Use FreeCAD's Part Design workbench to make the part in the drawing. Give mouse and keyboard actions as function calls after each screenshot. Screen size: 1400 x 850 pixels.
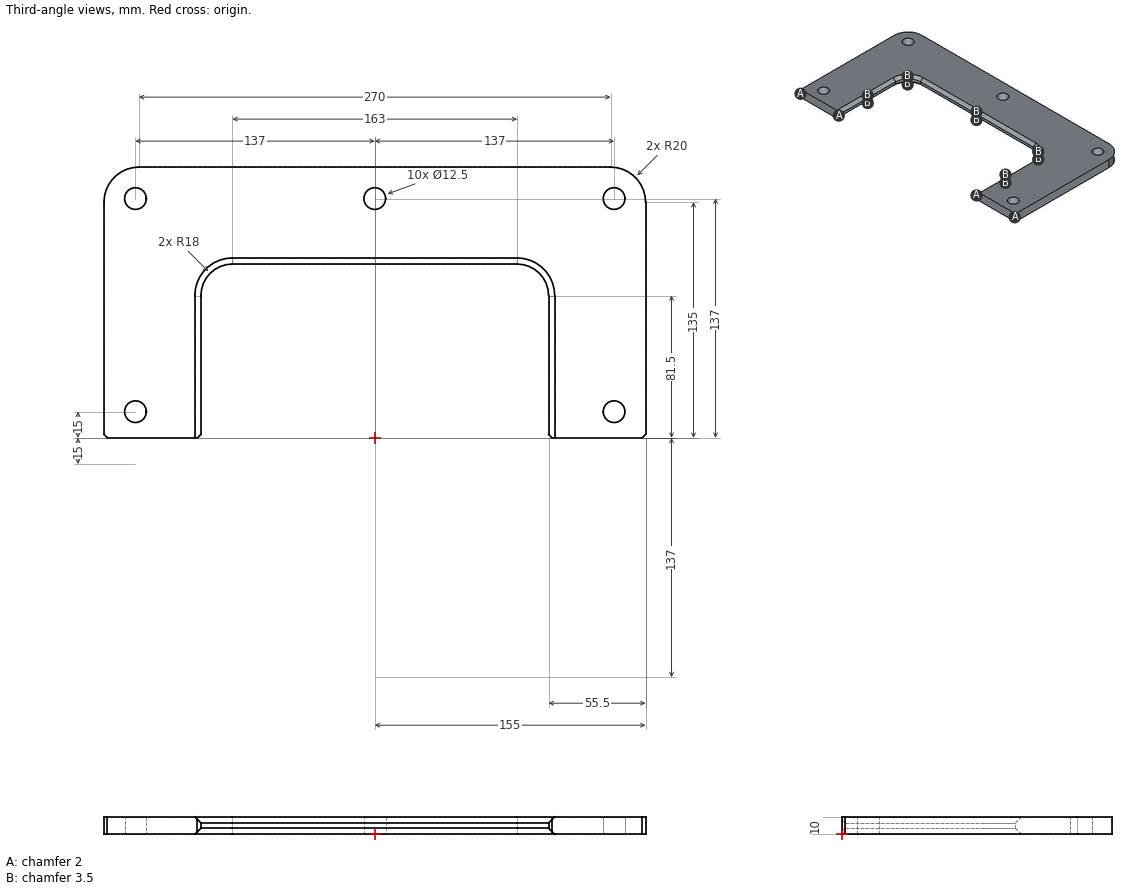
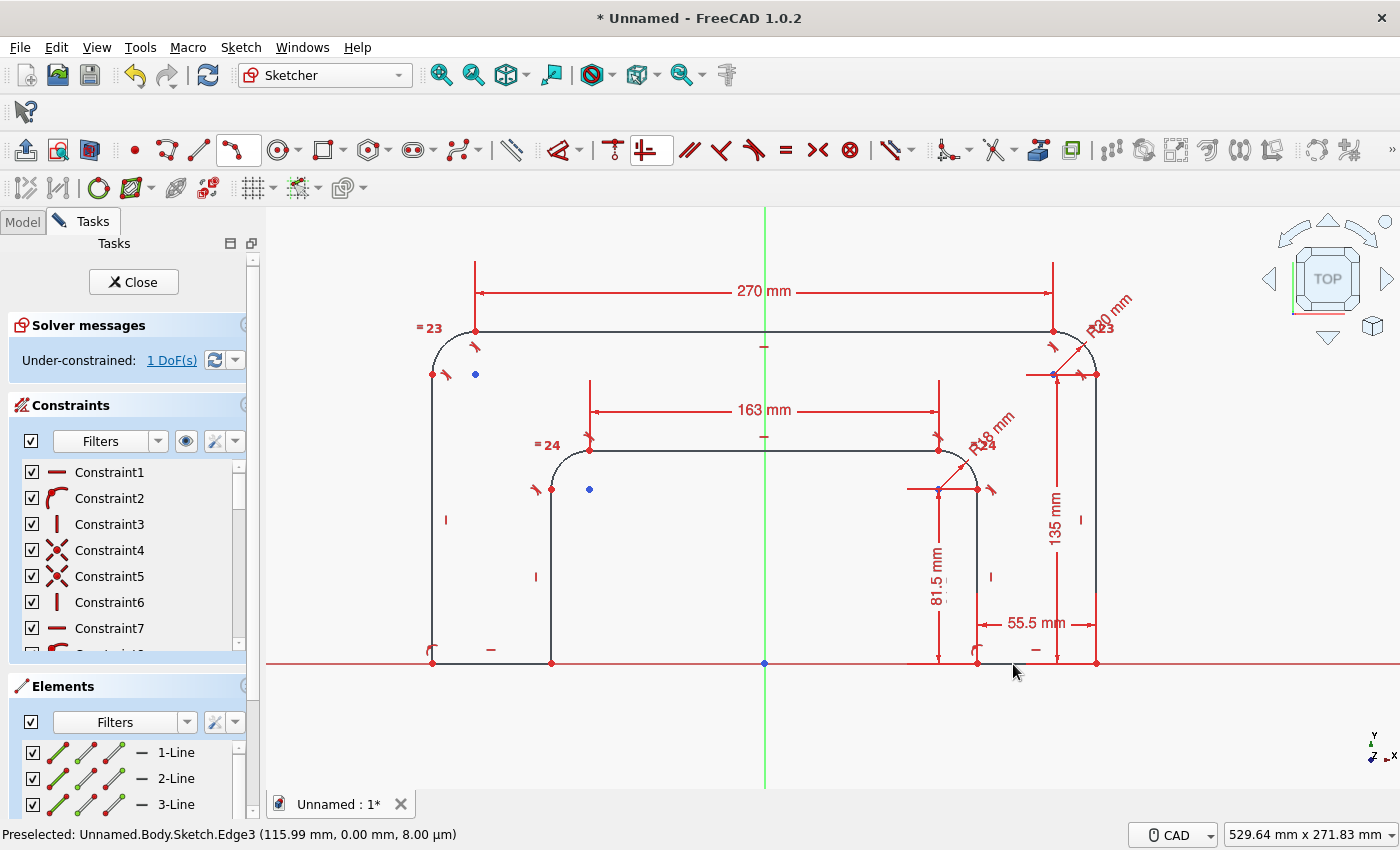
click(1096, 664)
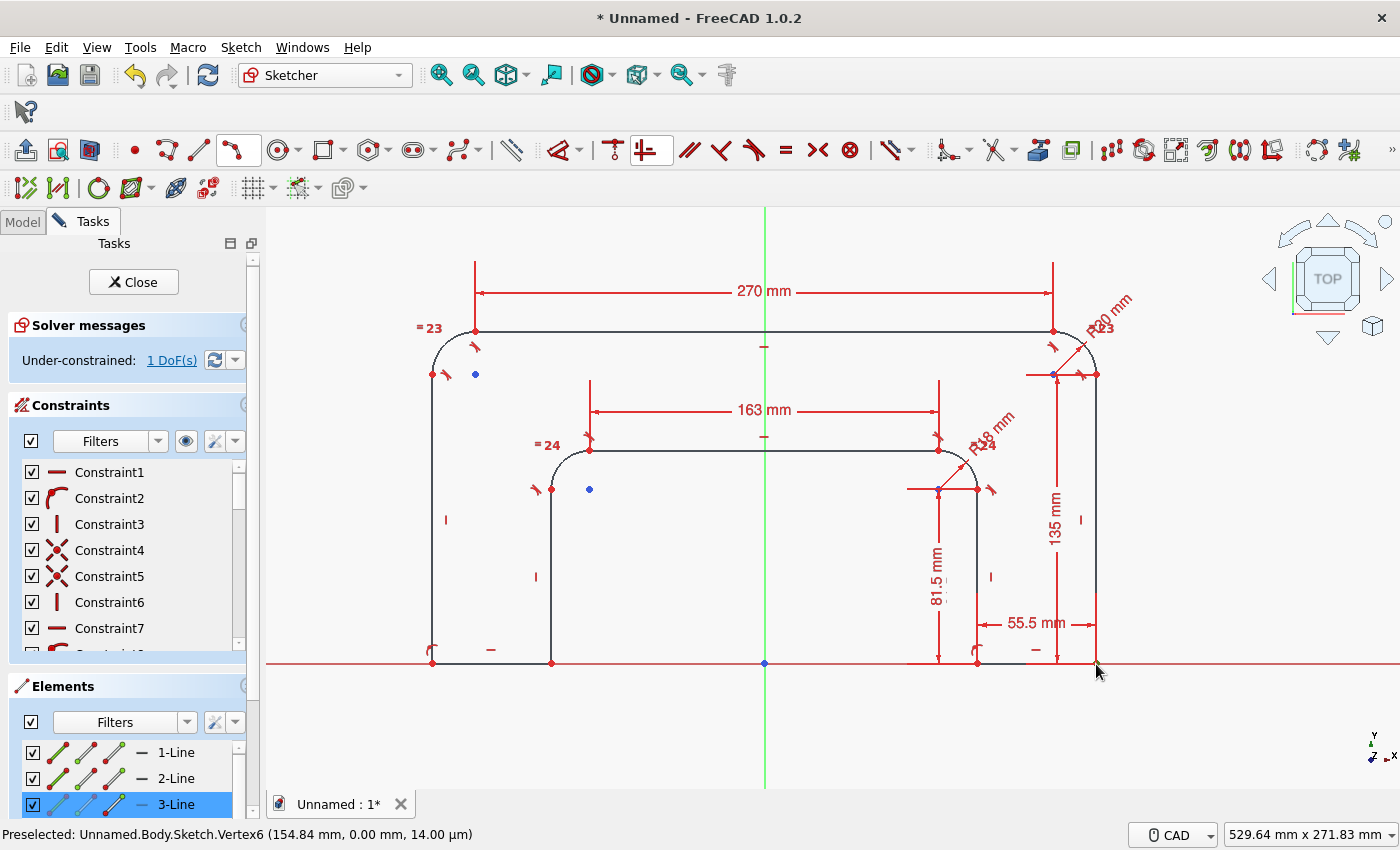
key(l)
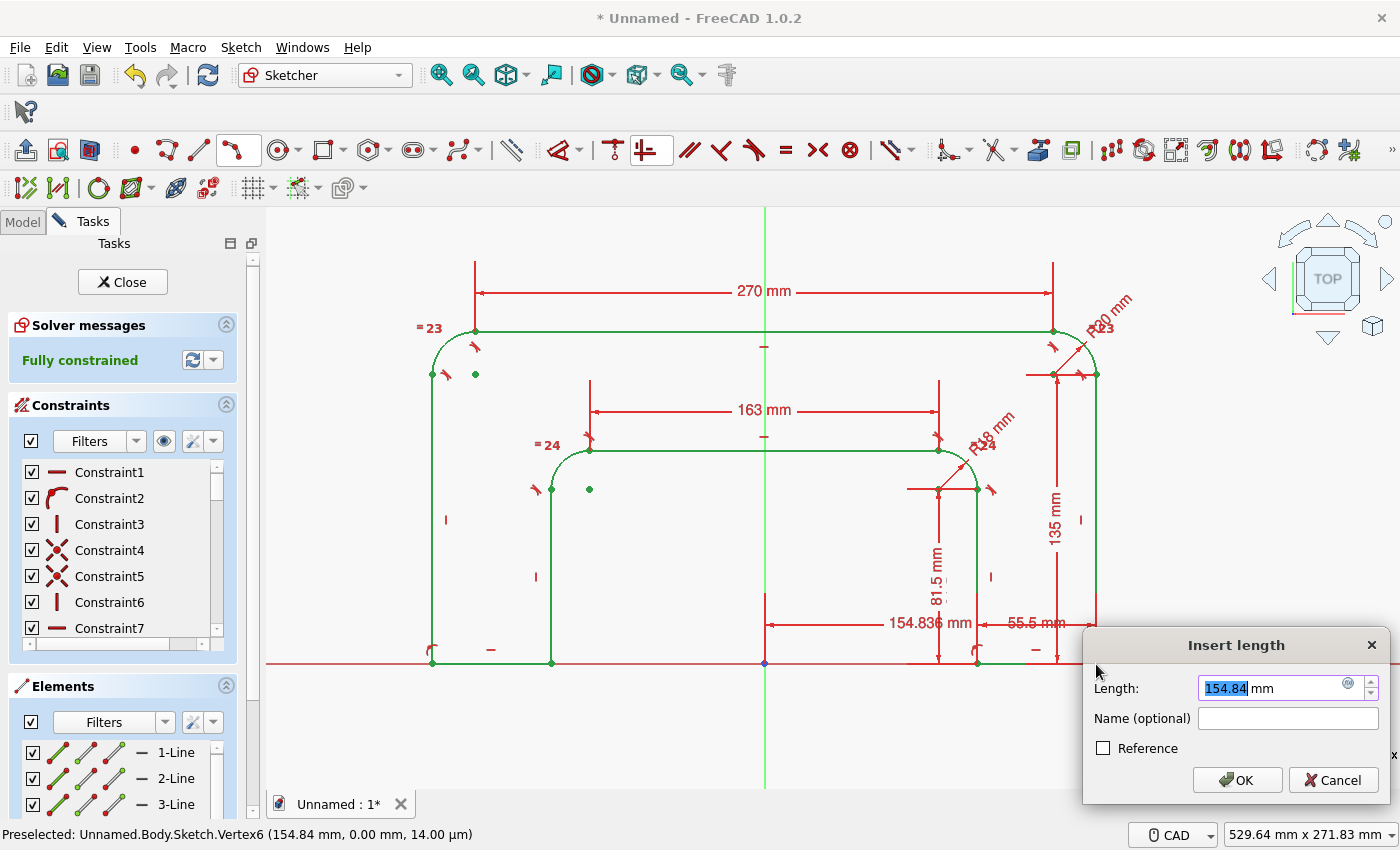
text(155)
key(Return)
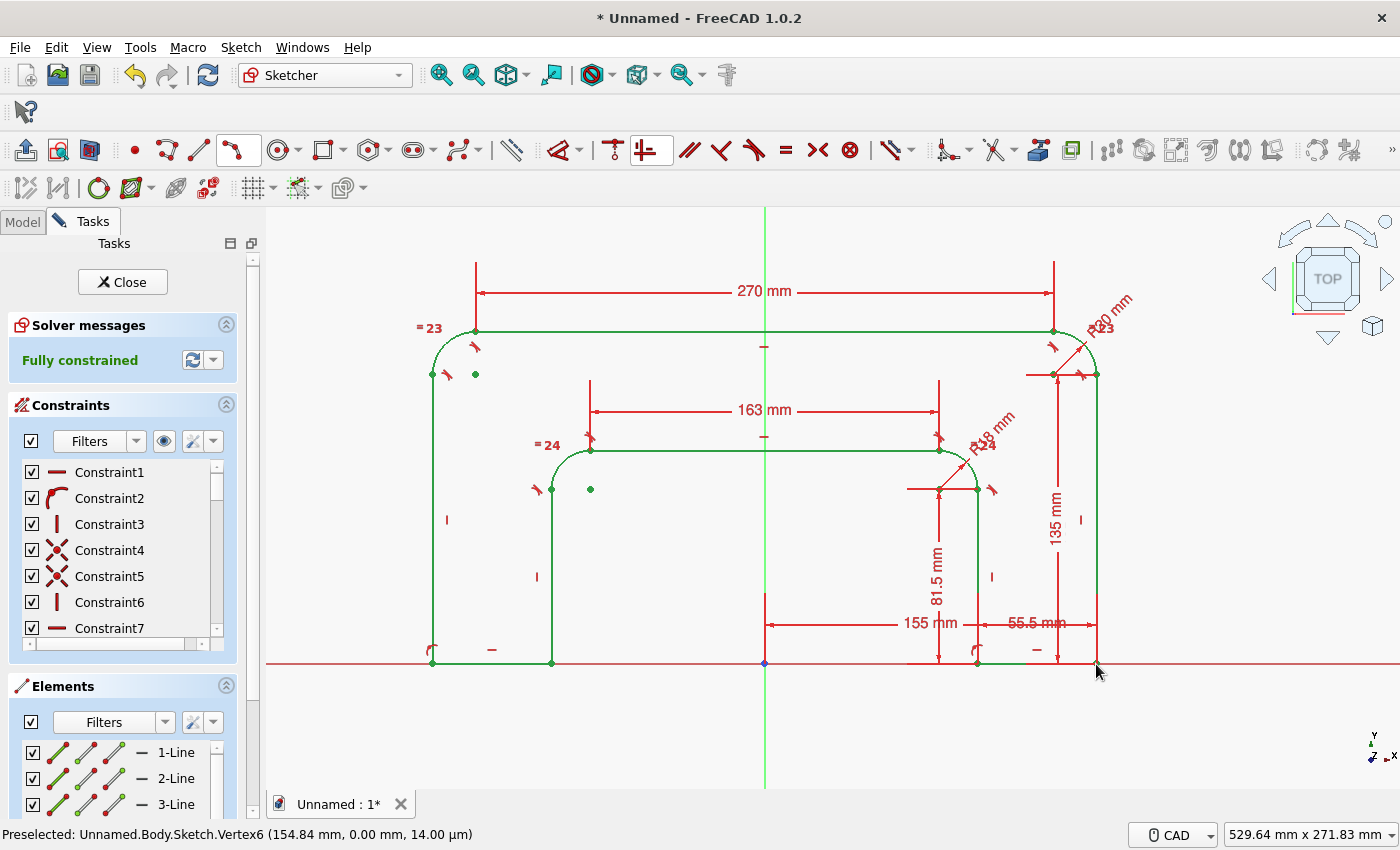
click(123, 282)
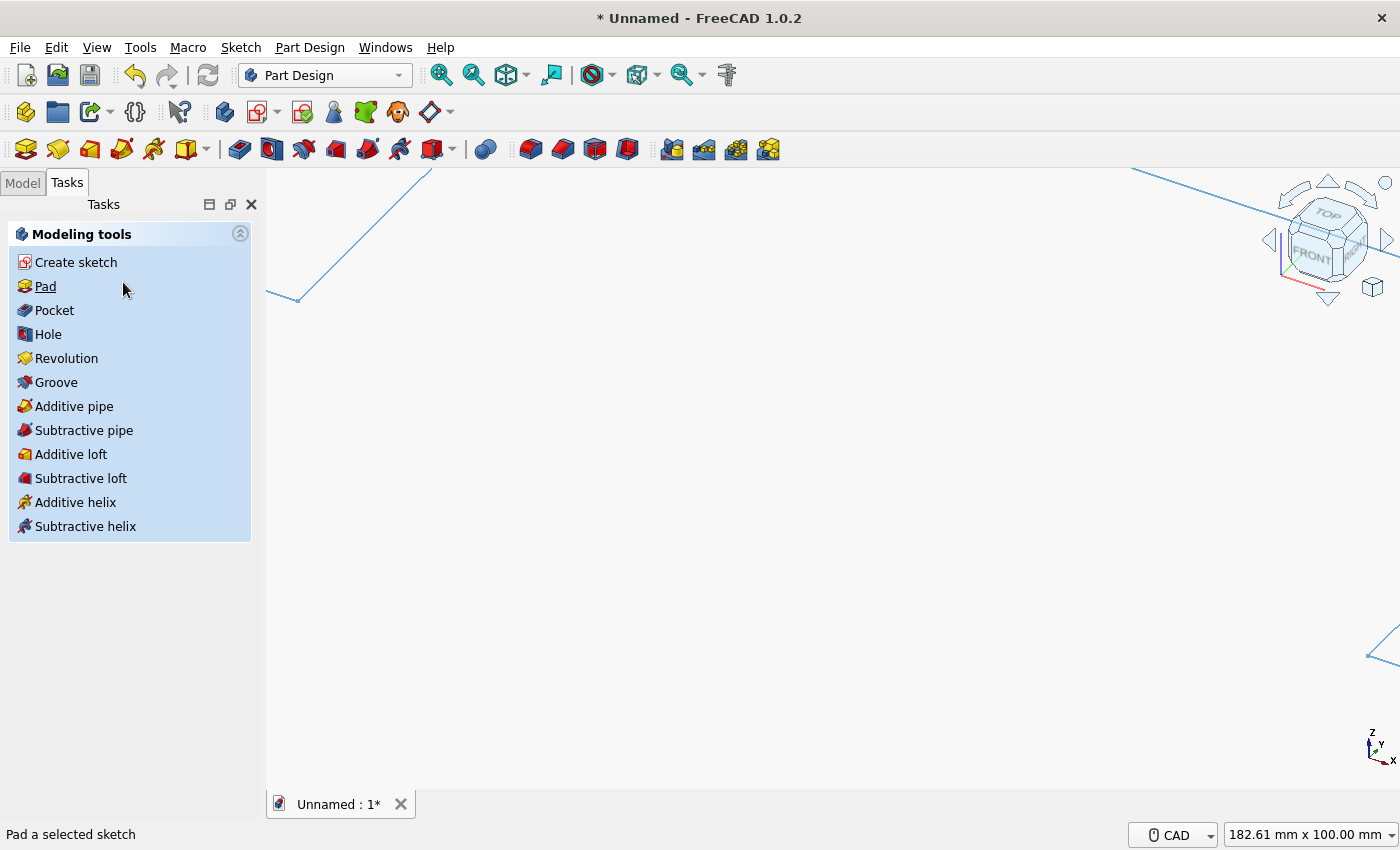
click(26, 150)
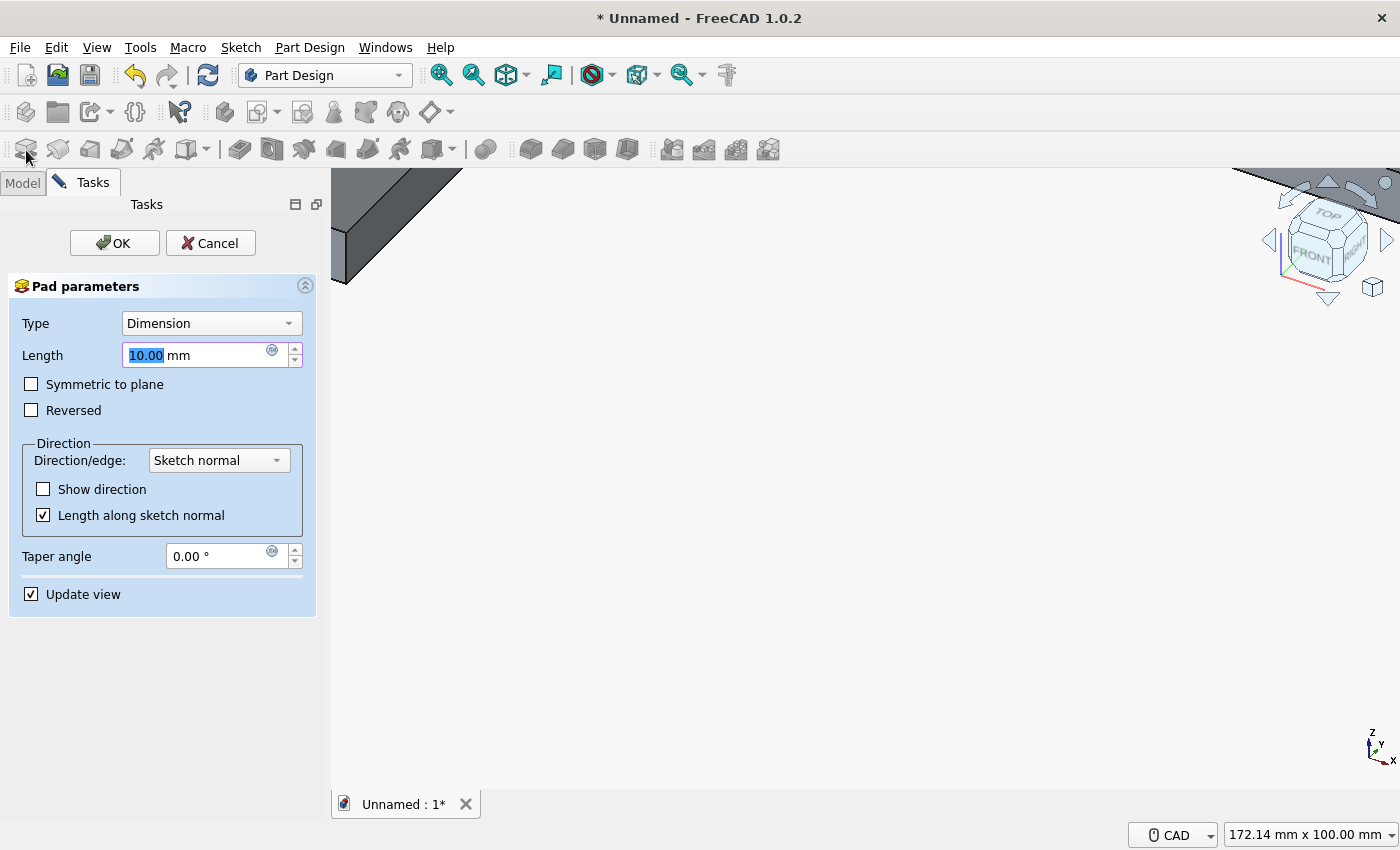
text(10)
key(Tab)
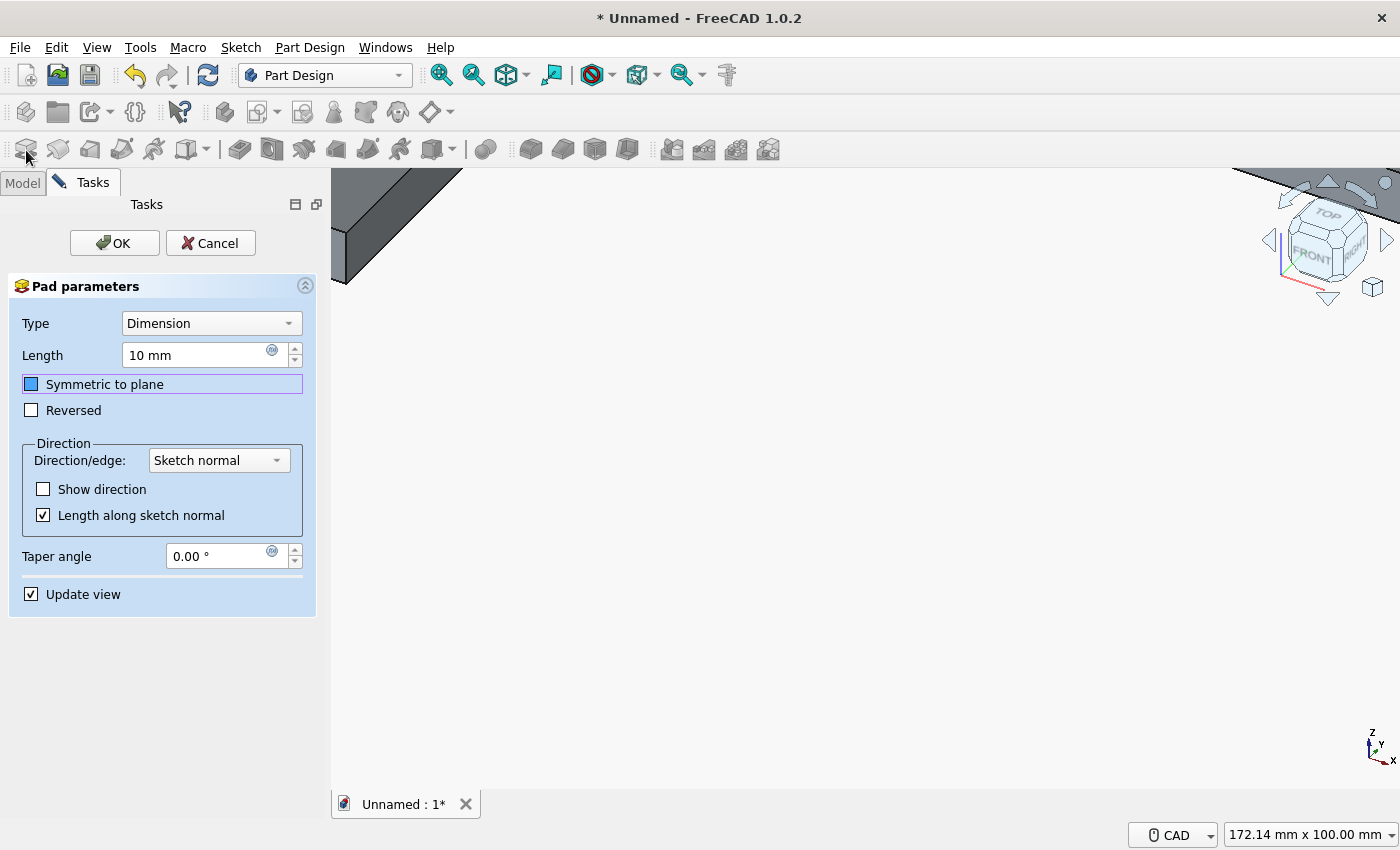
click(115, 243)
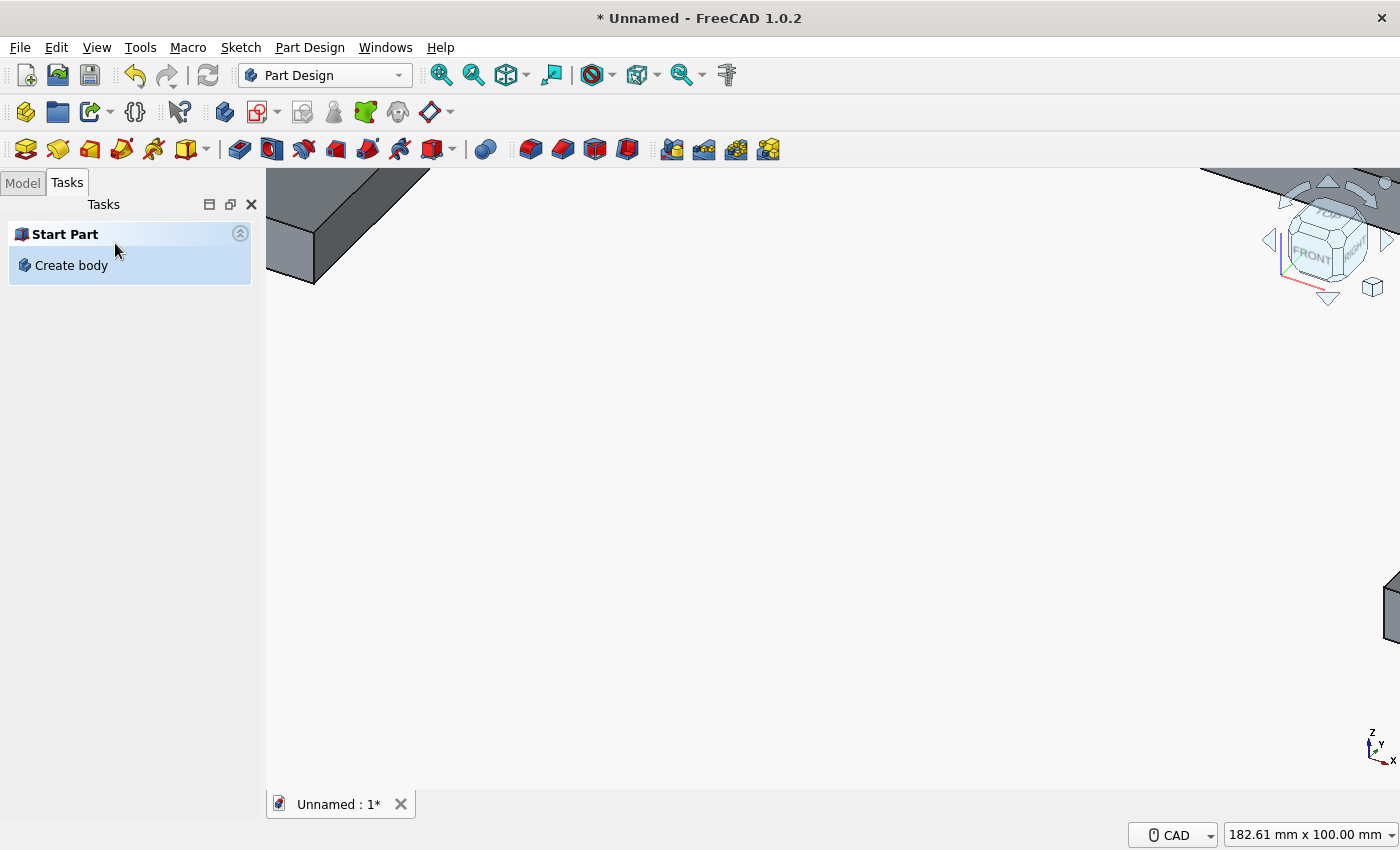
key(v)
key(f)